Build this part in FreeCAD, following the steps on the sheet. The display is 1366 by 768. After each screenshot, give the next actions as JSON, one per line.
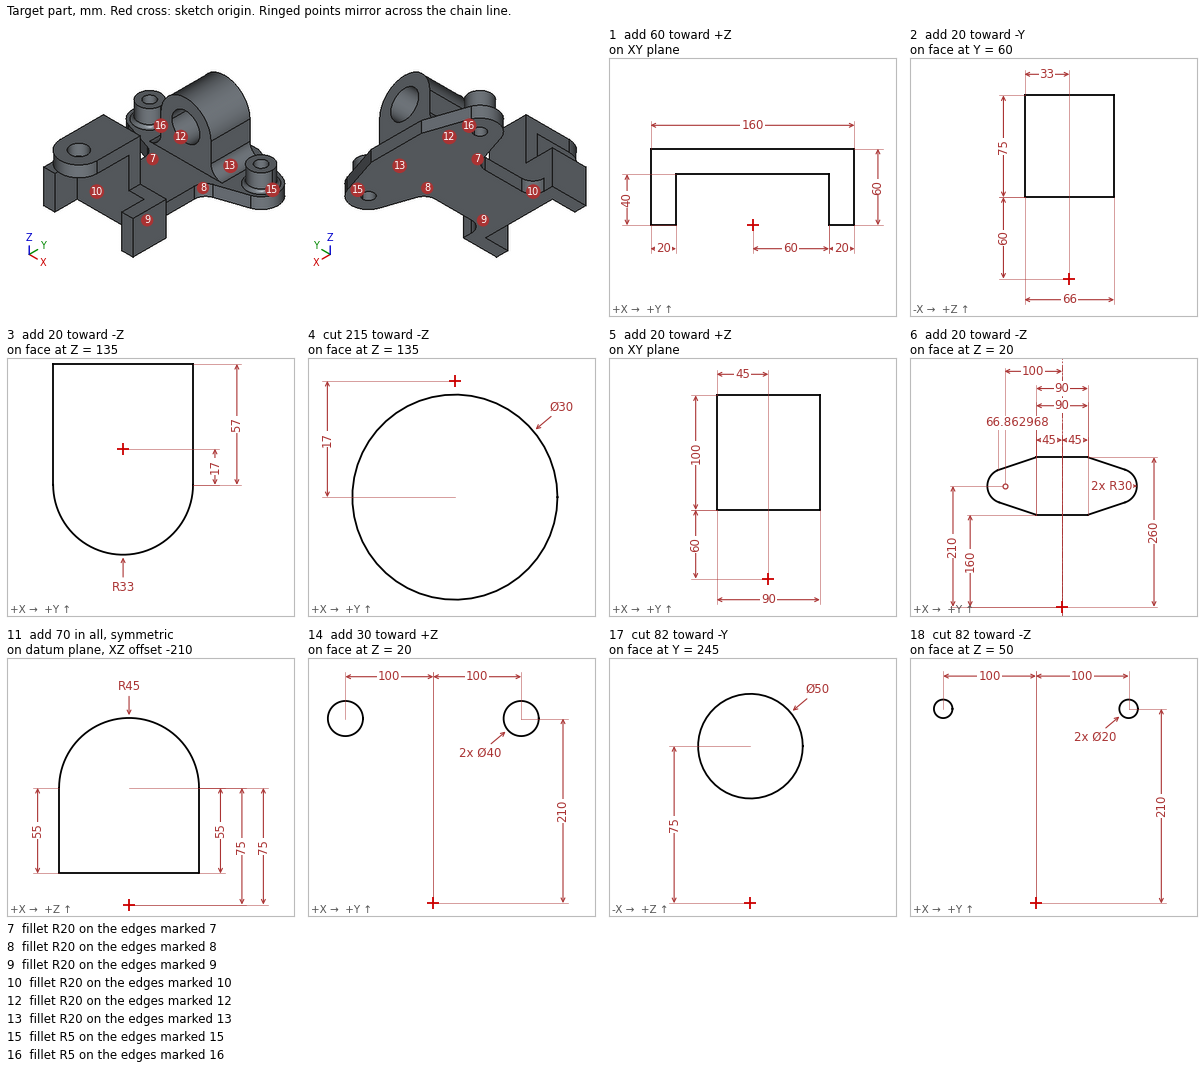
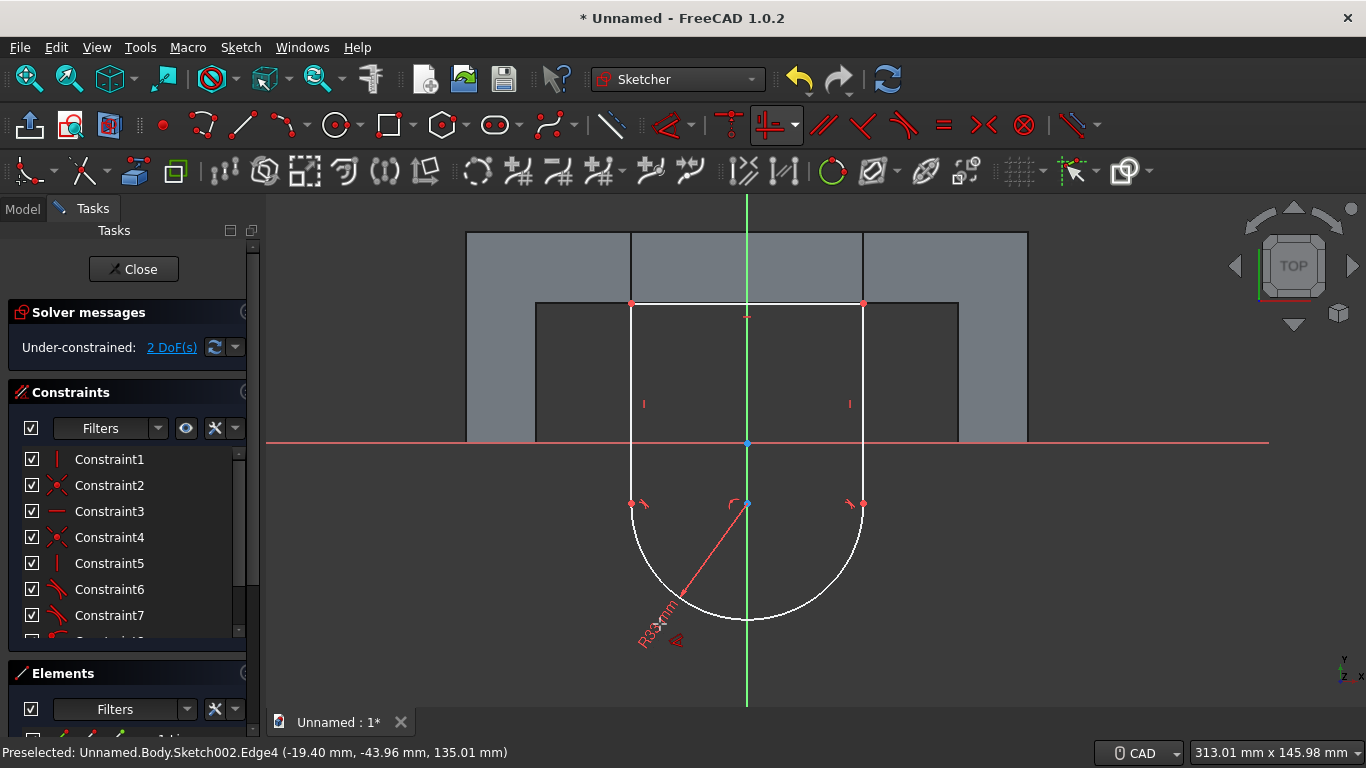
{"action": "left_click", "coordinate": [863, 444]}
{"action": "left_click", "coordinate": [897, 404]}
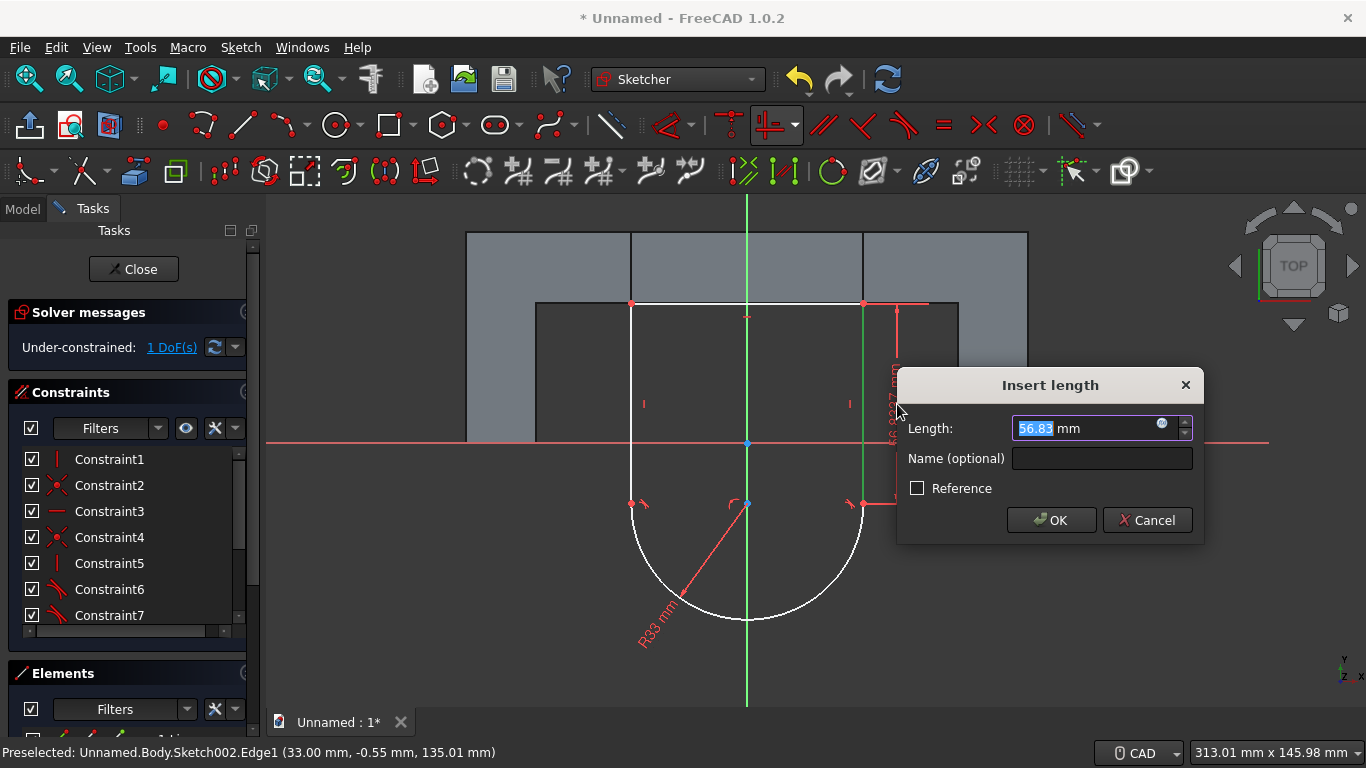
{"action": "type", "text": "57"}
{"action": "key", "text": "Return"}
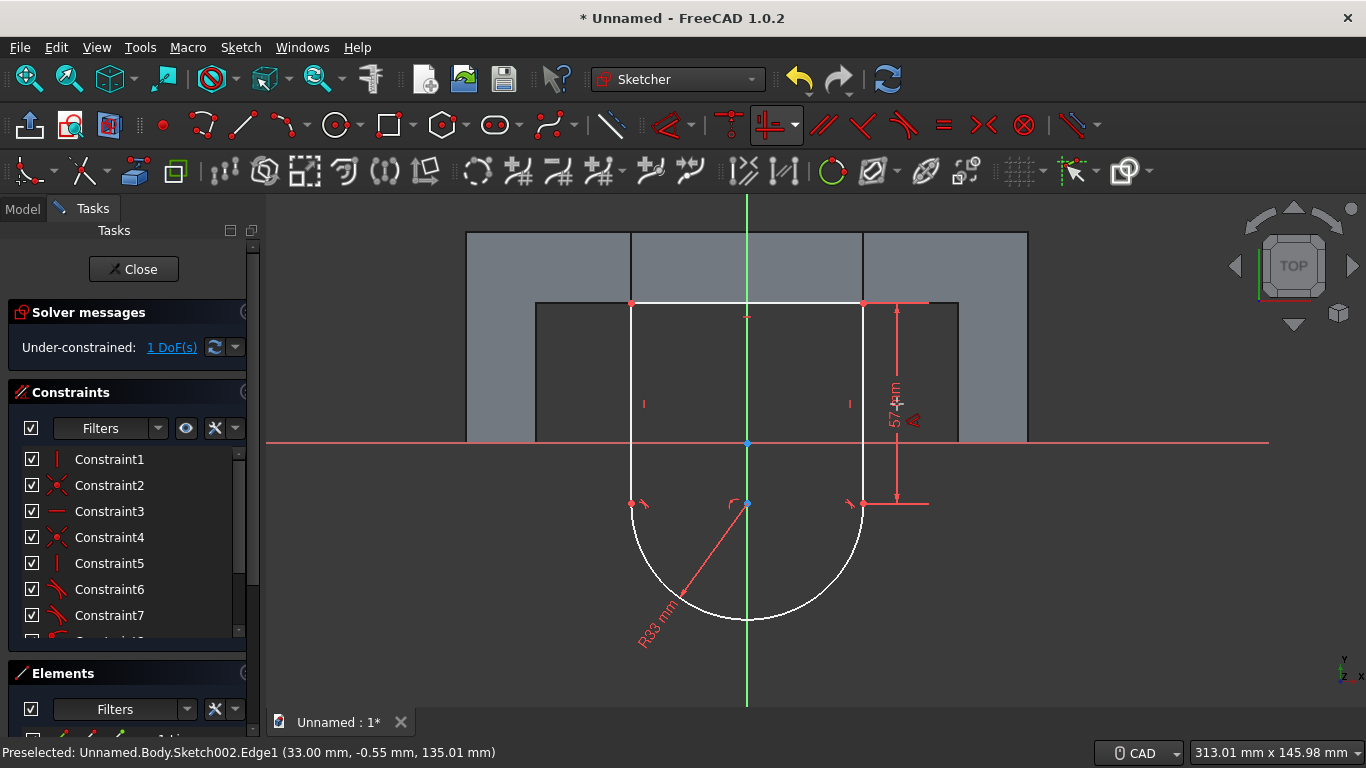
{"action": "left_click", "coordinate": [863, 504]}
{"action": "left_click", "coordinate": [897, 473]}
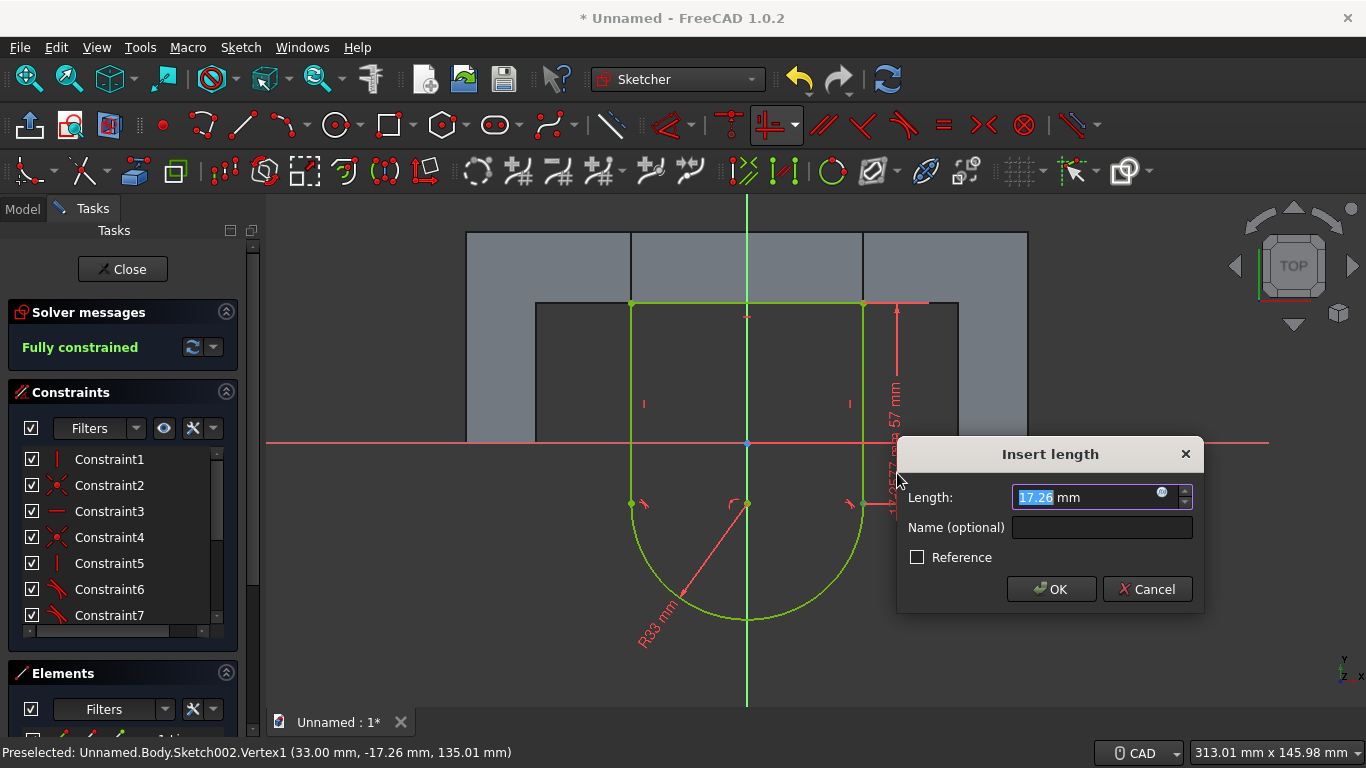
{"action": "type", "text": "17"}
{"action": "key", "text": "Return"}
{"action": "key", "text": "Escape"}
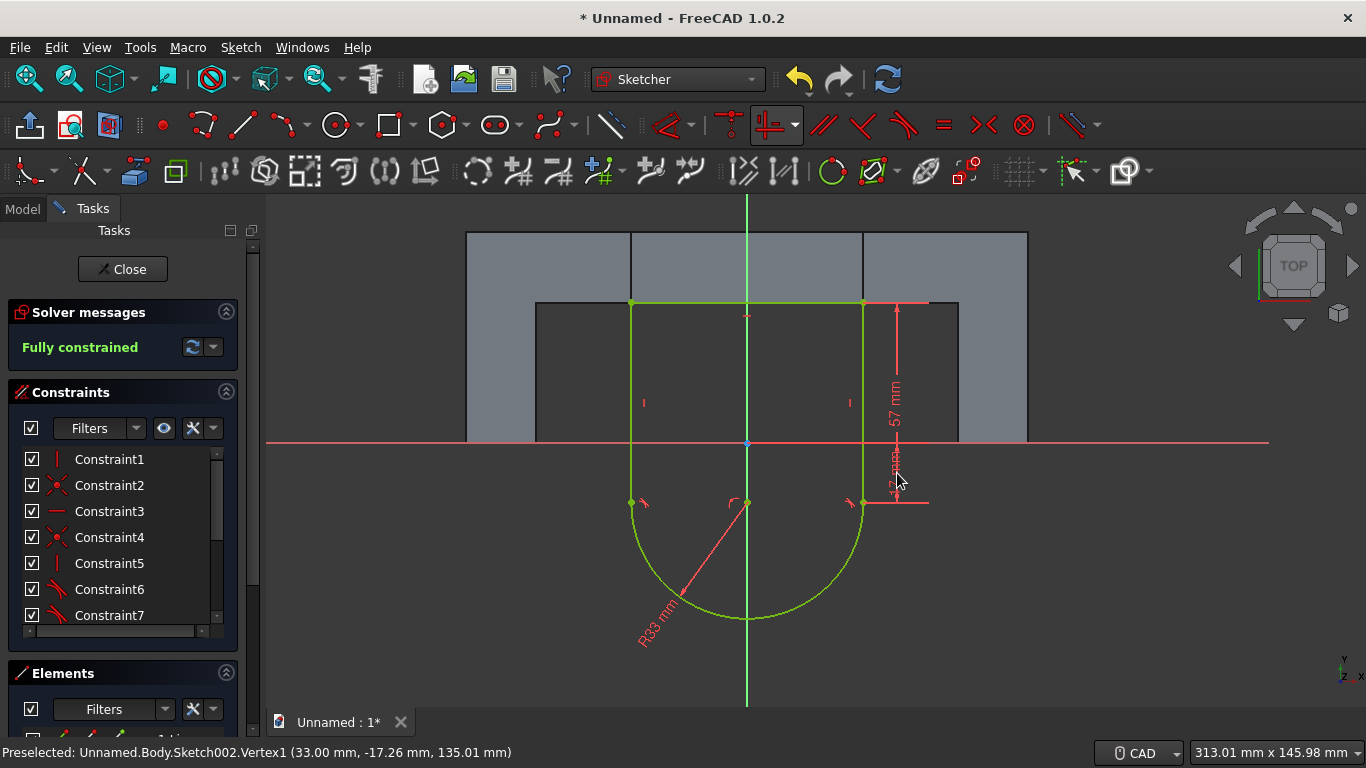
{"action": "left_click", "coordinate": [123, 269]}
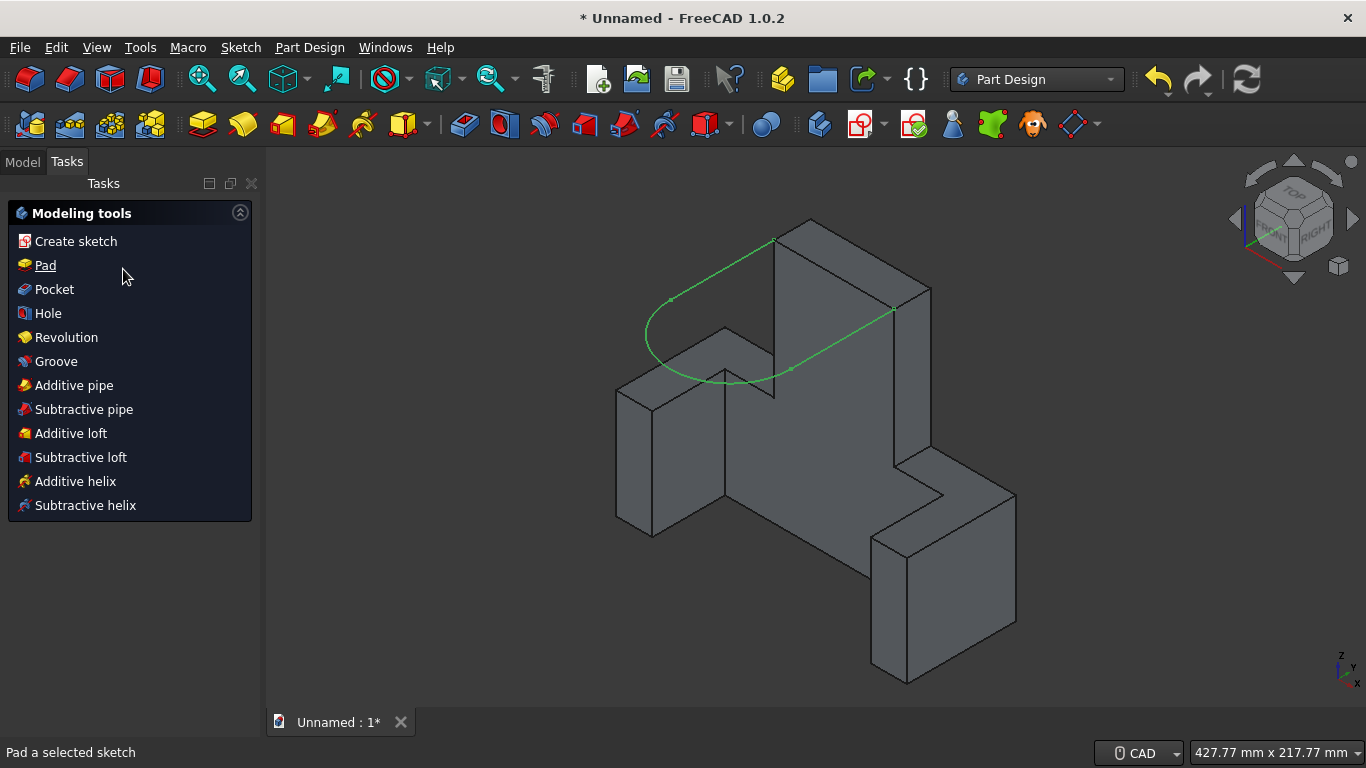
{"action": "left_click", "coordinate": [204, 124]}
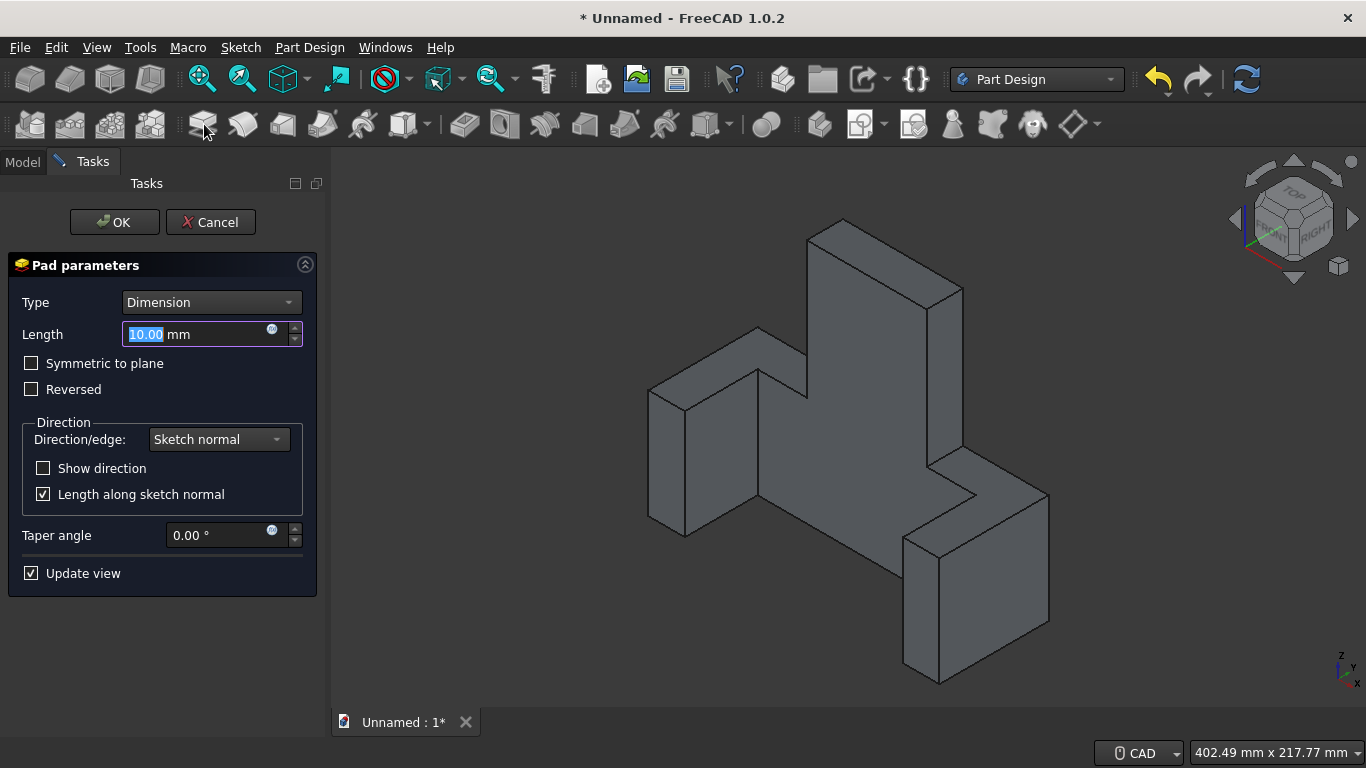
{"action": "type", "text": "20"}
{"action": "key", "text": "Tab"}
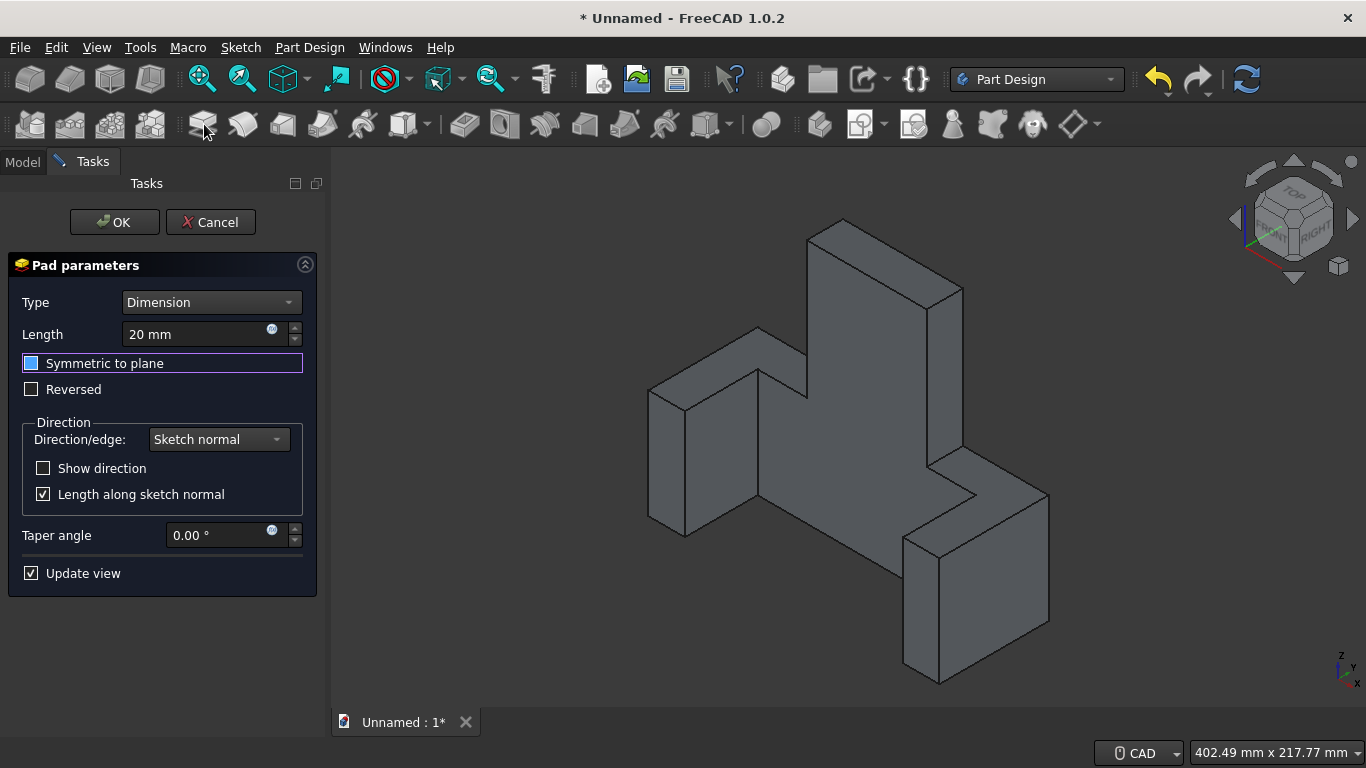
{"action": "left_click", "coordinate": [30, 389]}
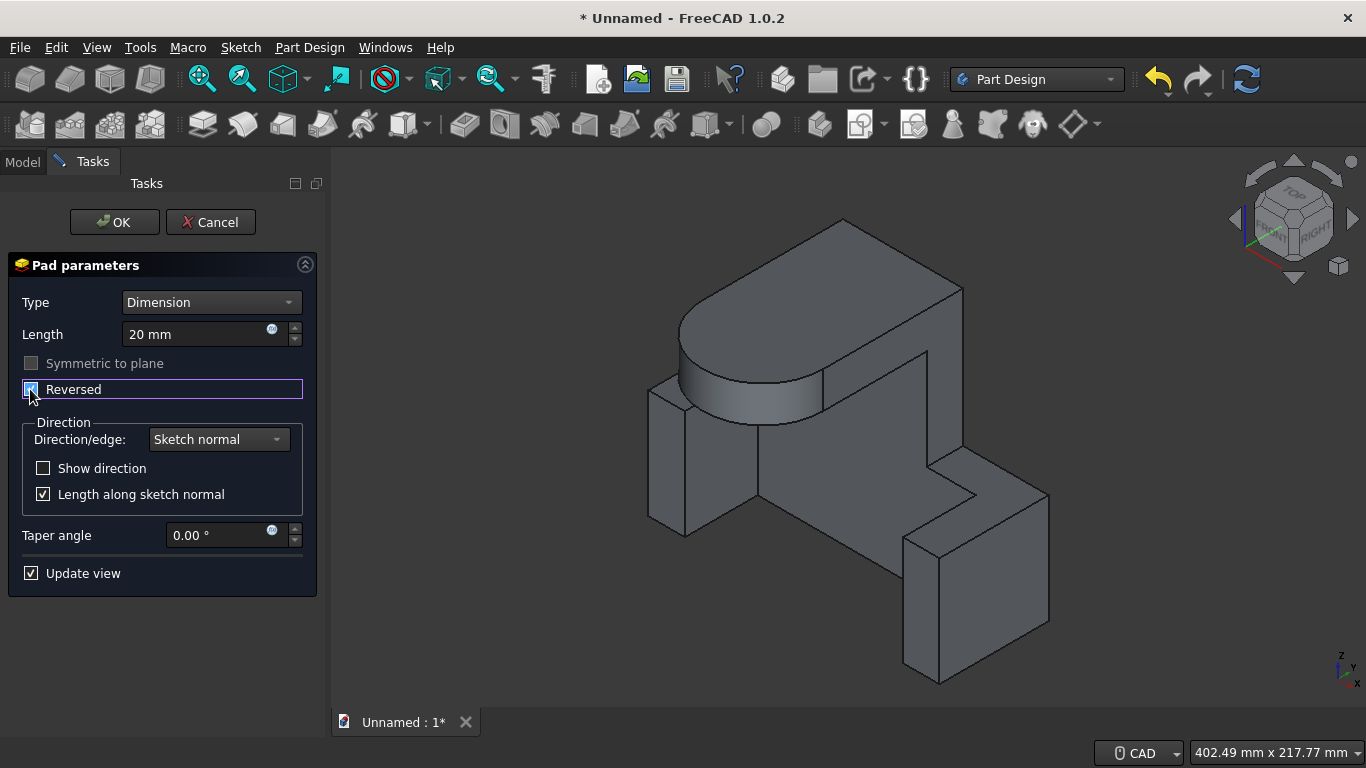
{"action": "left_click", "coordinate": [115, 222]}